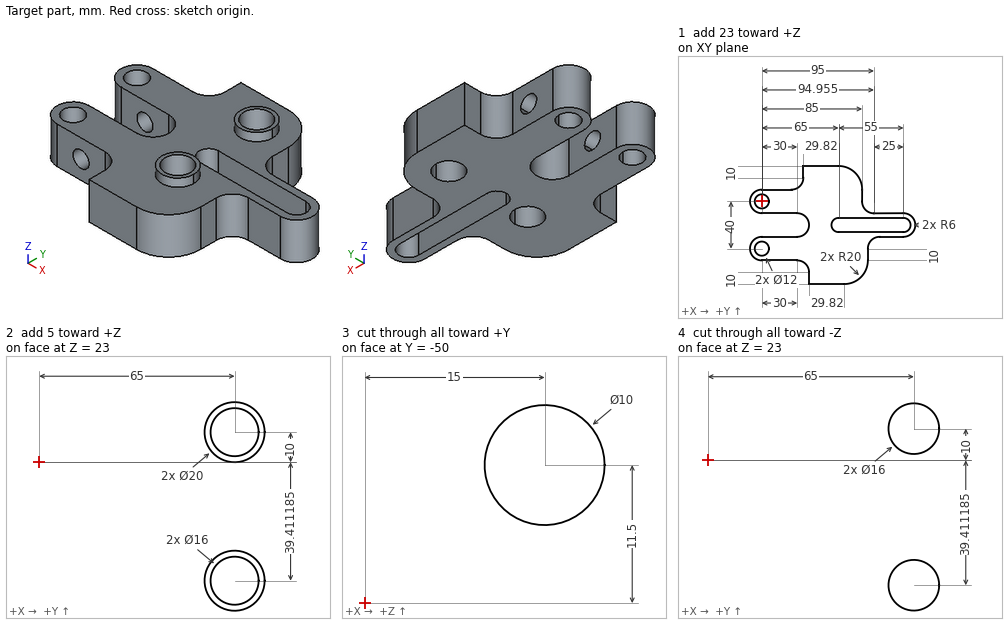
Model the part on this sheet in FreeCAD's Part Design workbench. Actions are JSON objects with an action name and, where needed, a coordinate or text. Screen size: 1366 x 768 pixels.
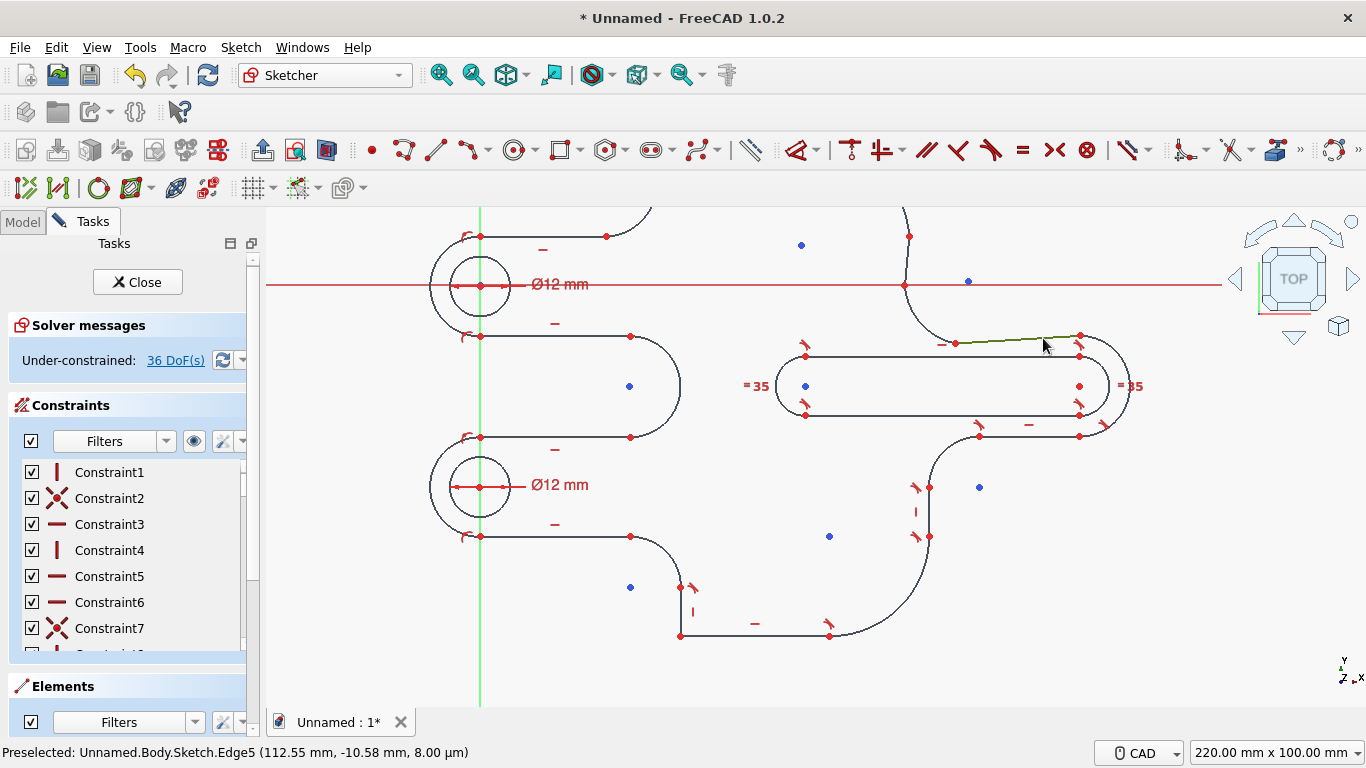
{"action": "left_click", "coordinate": [911, 309]}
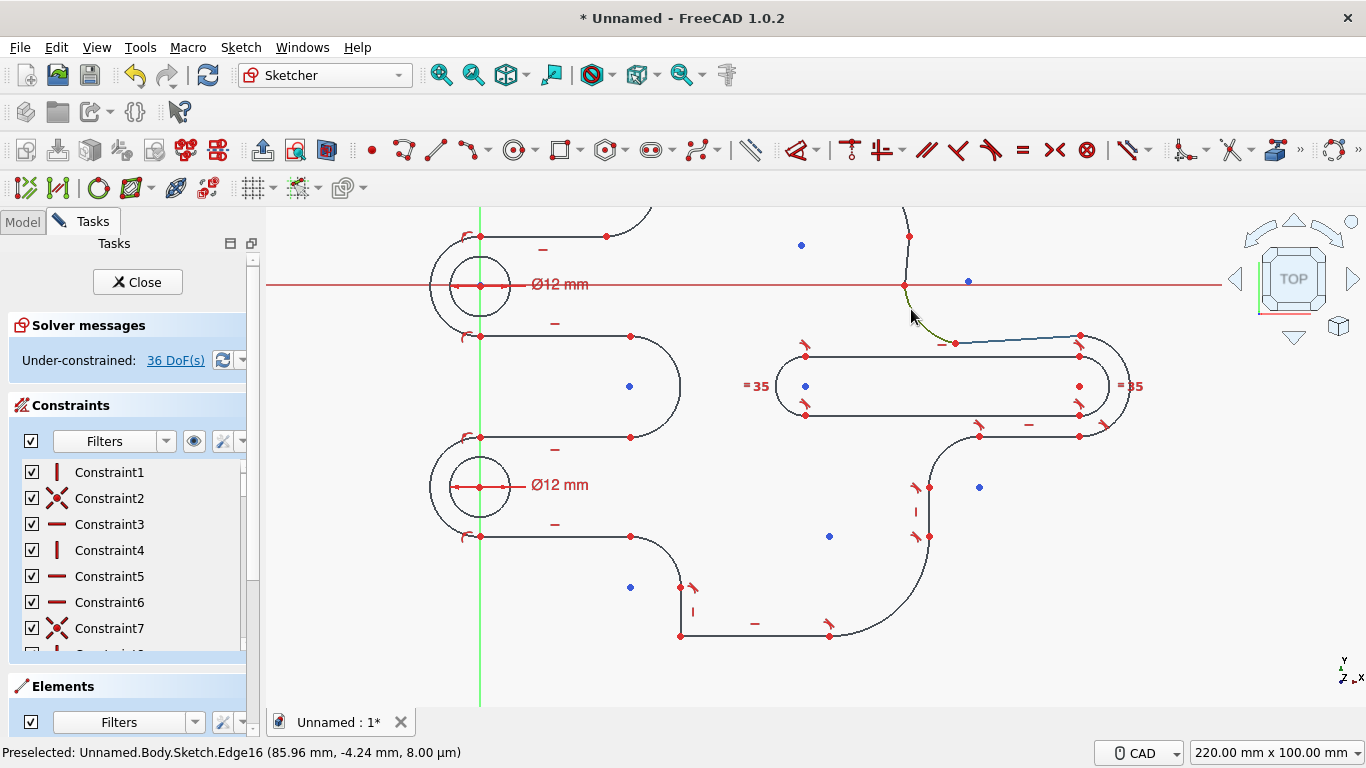
{"action": "left_click", "coordinate": [992, 150]}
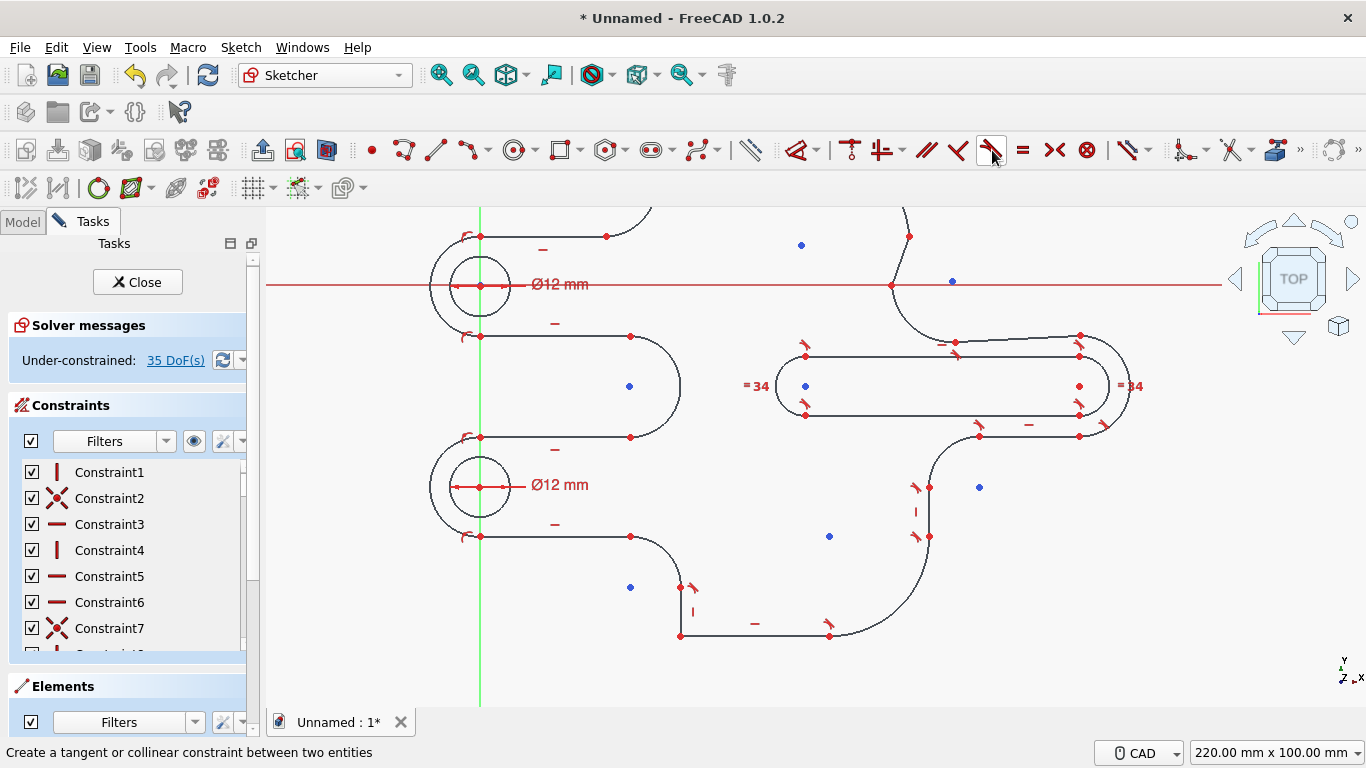
{"action": "left_click", "coordinate": [897, 271]}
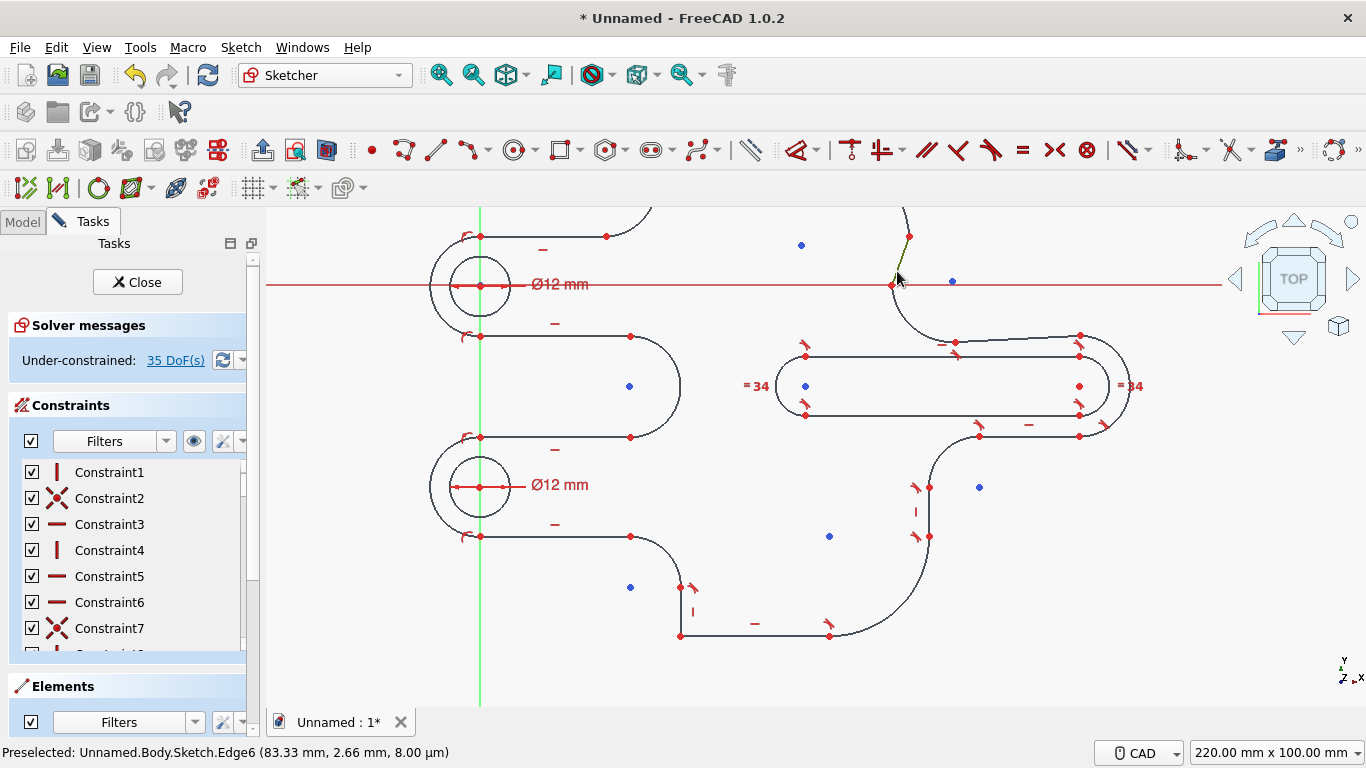
{"action": "left_click", "coordinate": [900, 312]}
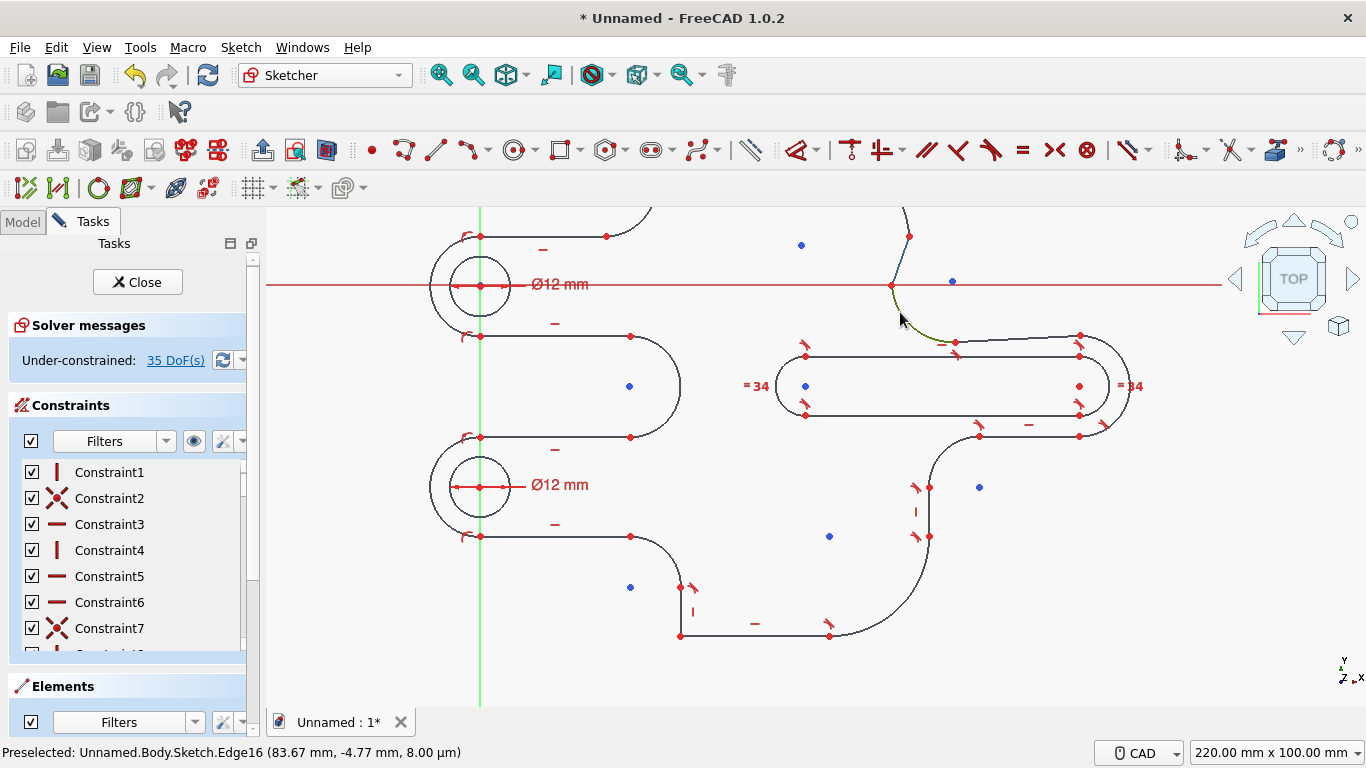
{"action": "left_click", "coordinate": [992, 150]}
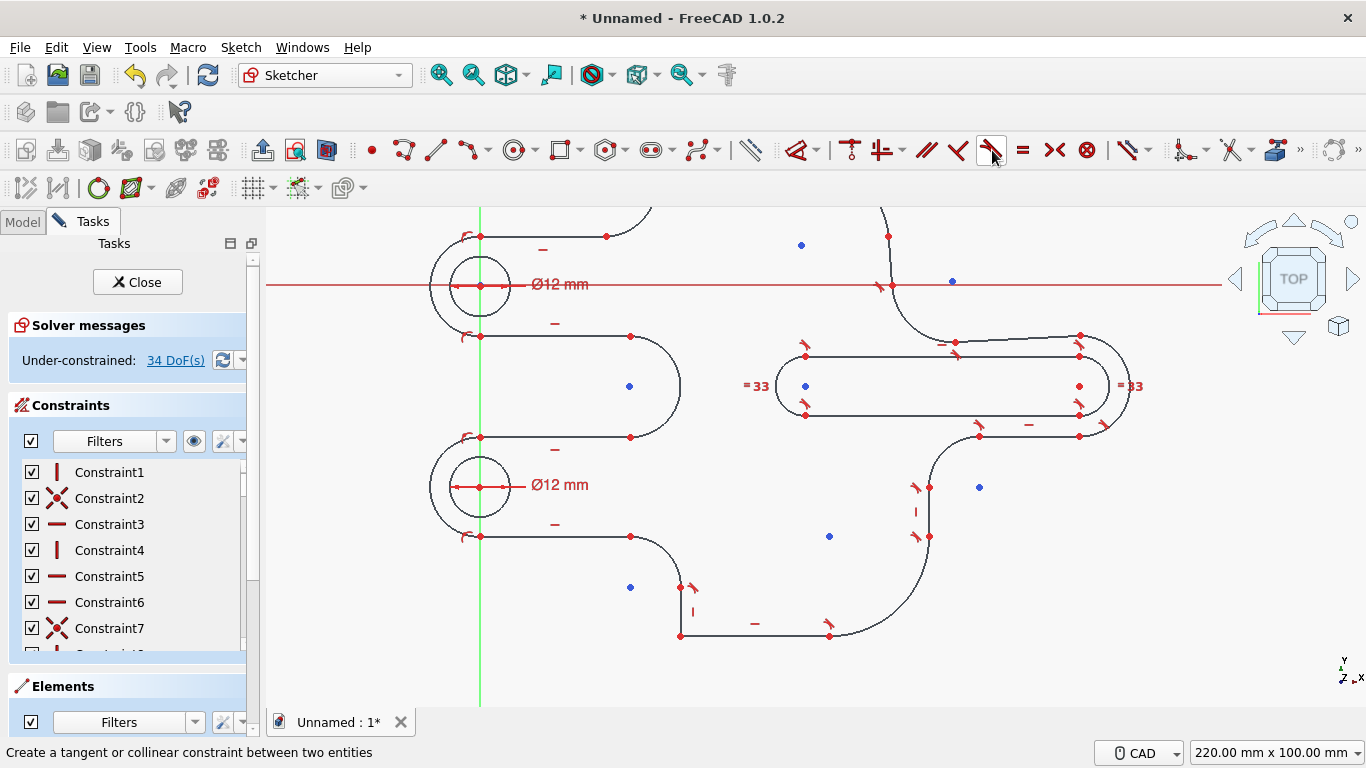
{"action": "left_click", "coordinate": [891, 271]}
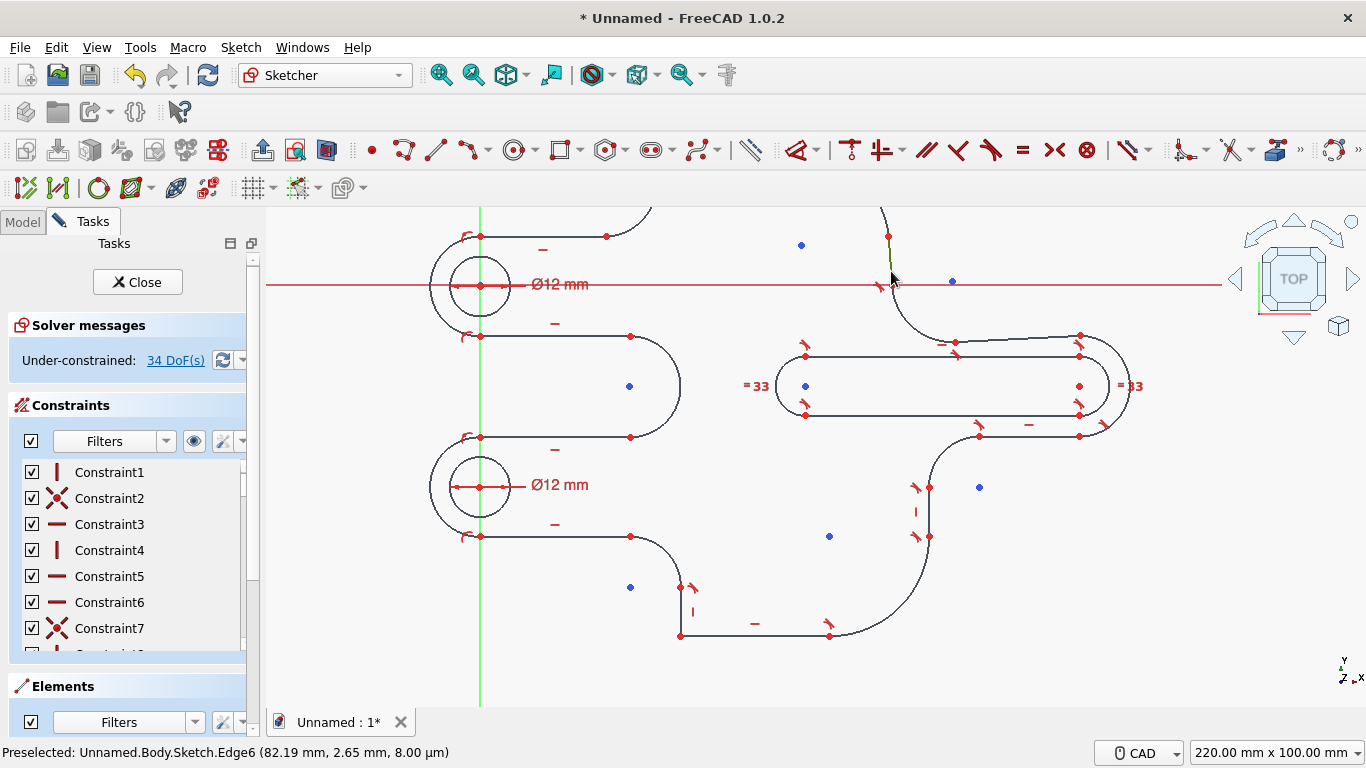
{"action": "scroll", "coordinate": [681, 603], "scroll_direction": "down", "scroll_amount": 2}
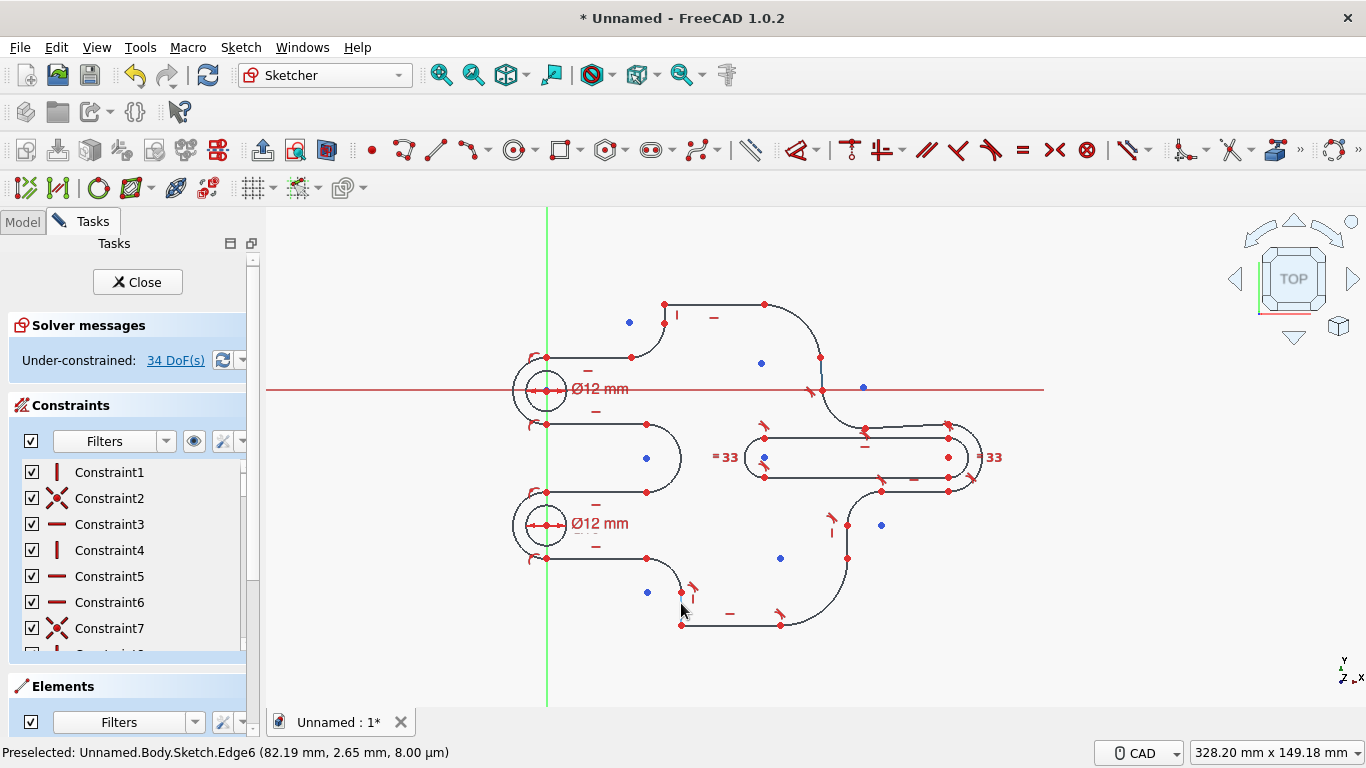
{"action": "left_click", "coordinate": [813, 334]}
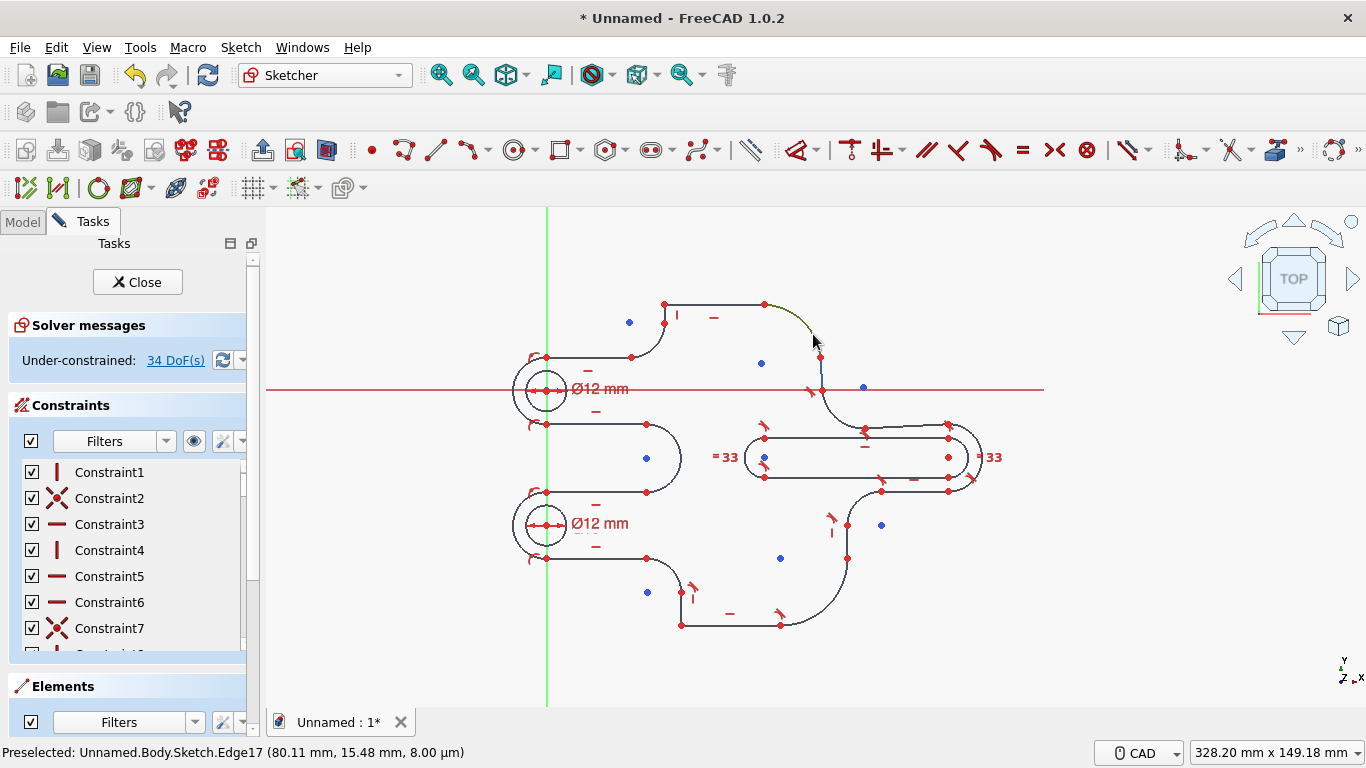
{"action": "left_click", "coordinate": [992, 150]}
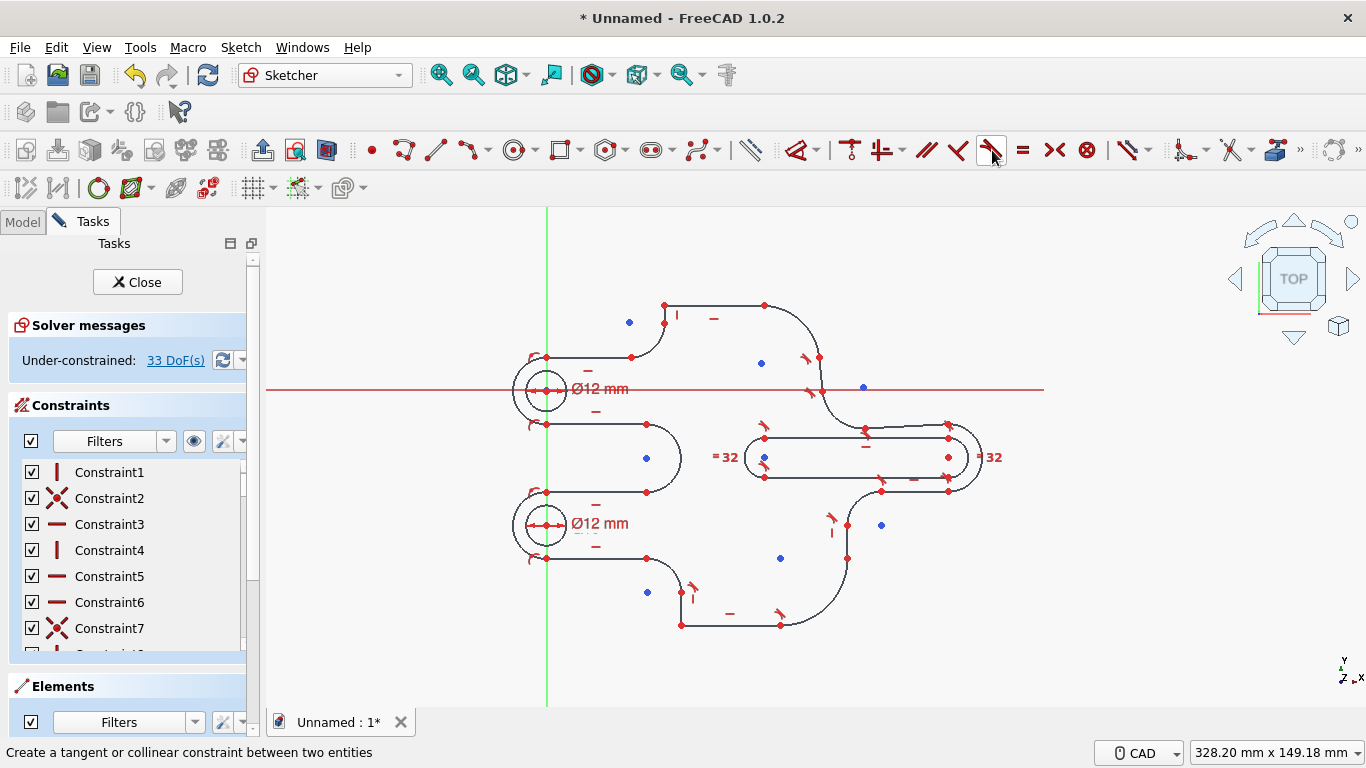
{"action": "left_click", "coordinate": [735, 306]}